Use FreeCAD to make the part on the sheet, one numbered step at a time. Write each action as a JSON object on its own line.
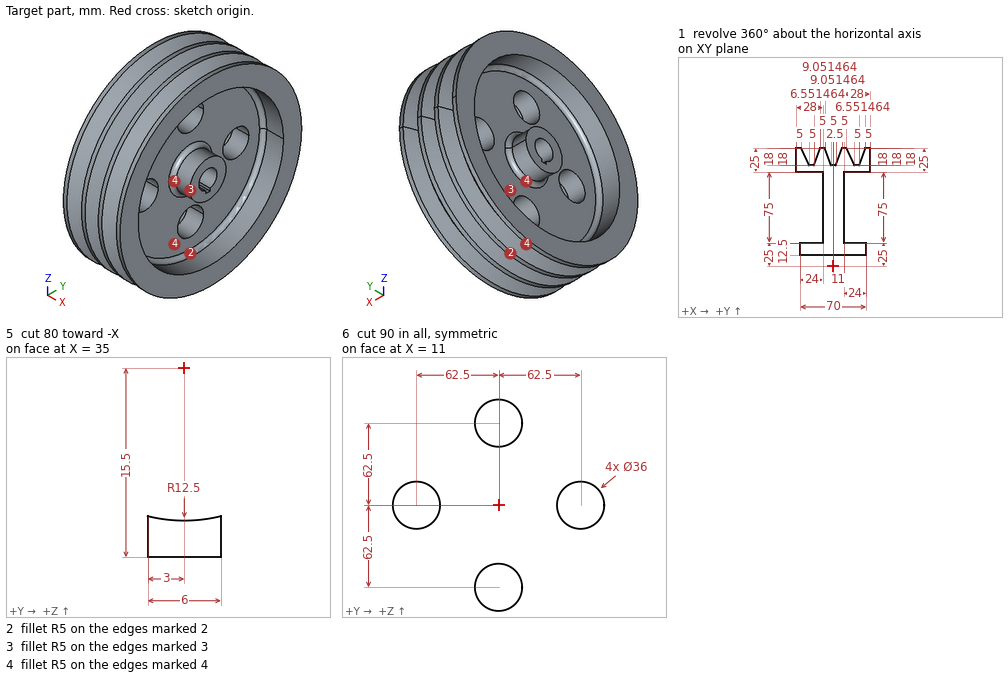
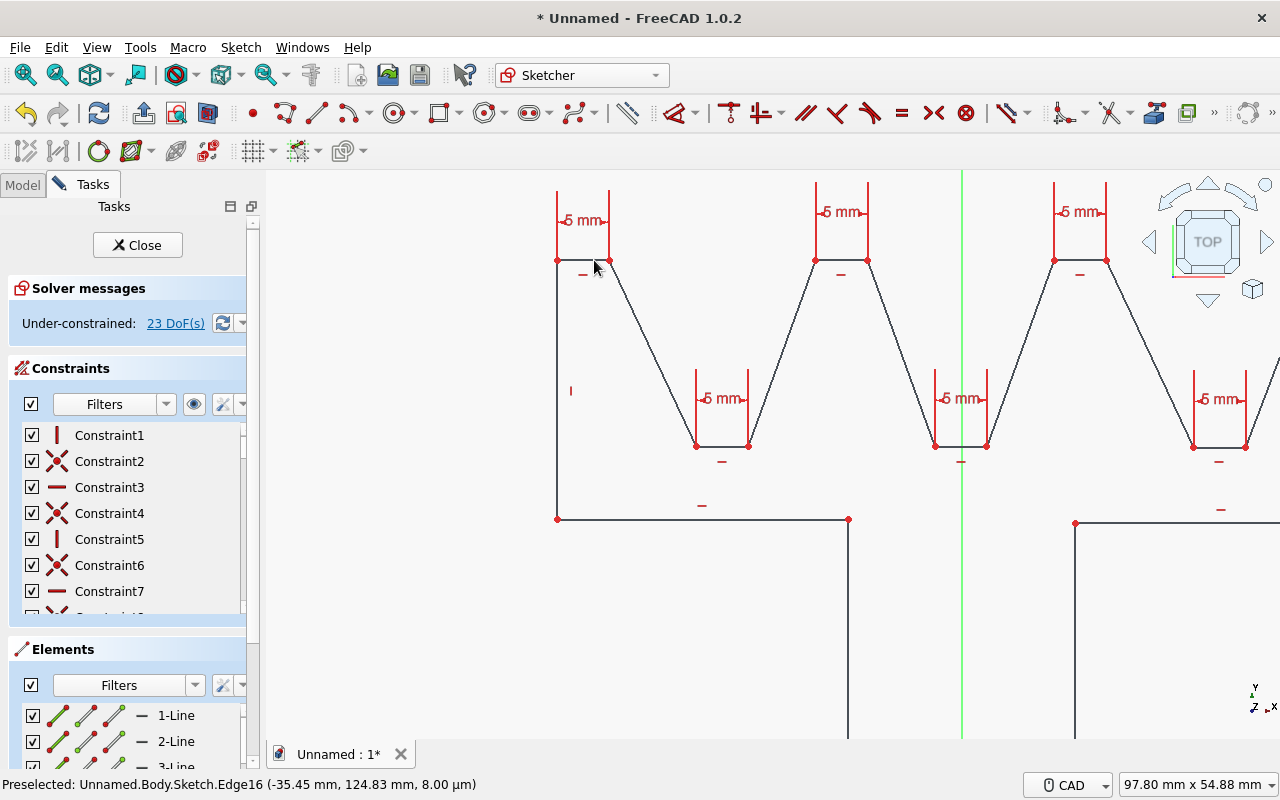
{"action": "scroll", "coordinate": [594, 260], "scroll_direction": "down", "scroll_amount": 6}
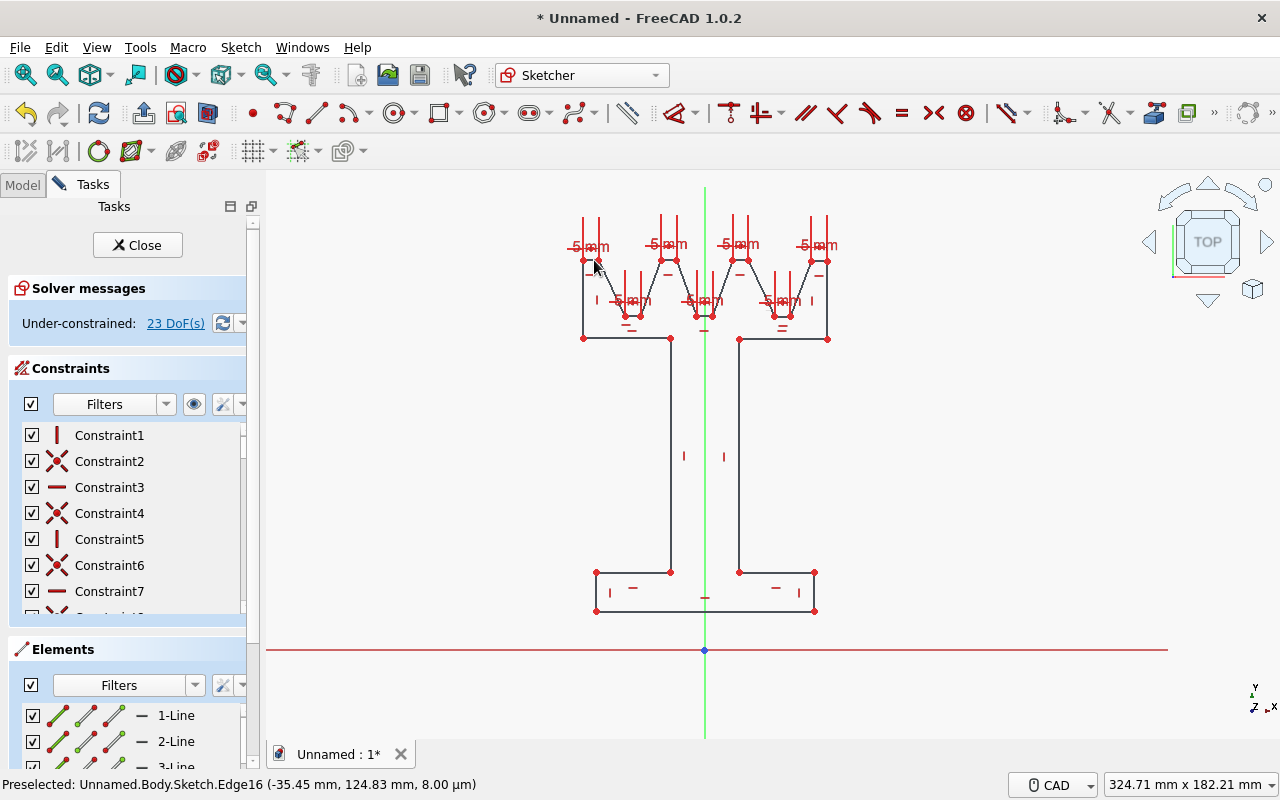
{"action": "left_click", "coordinate": [739, 386]}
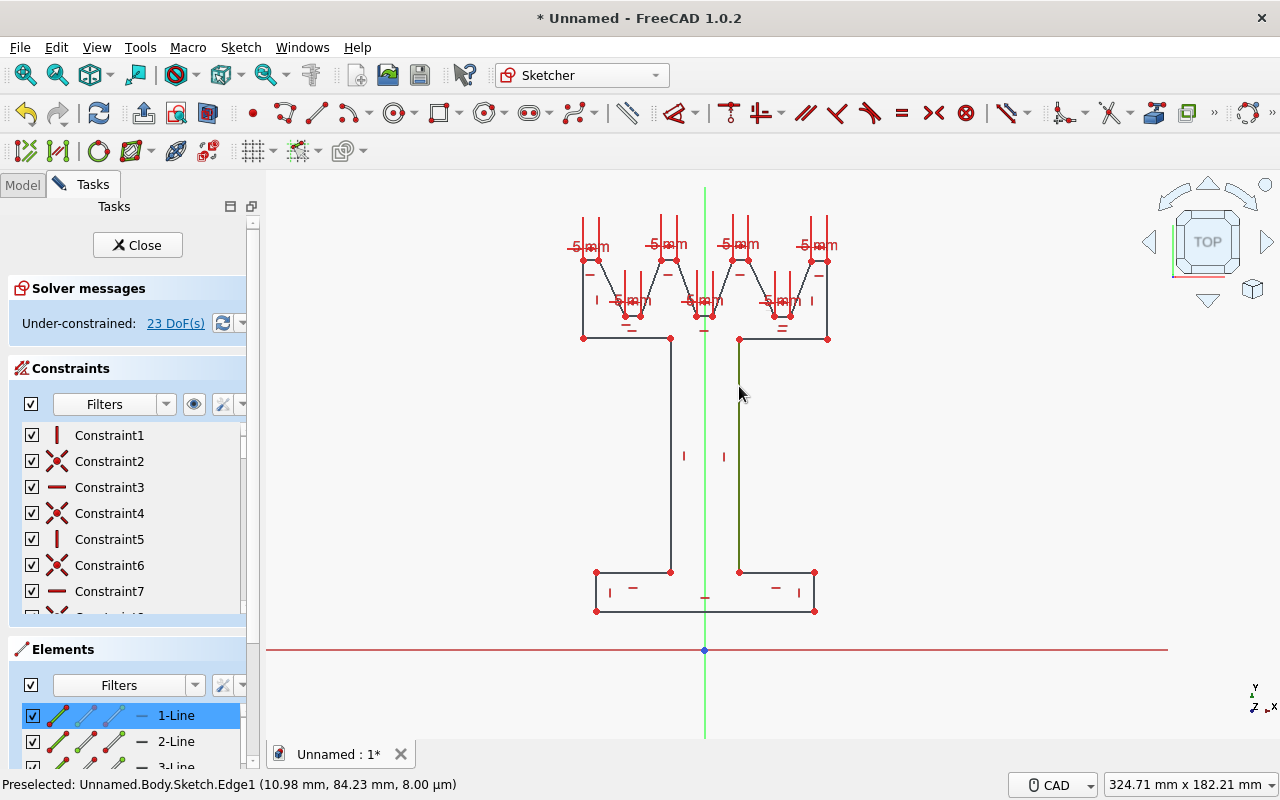
{"action": "left_click", "coordinate": [698, 114]}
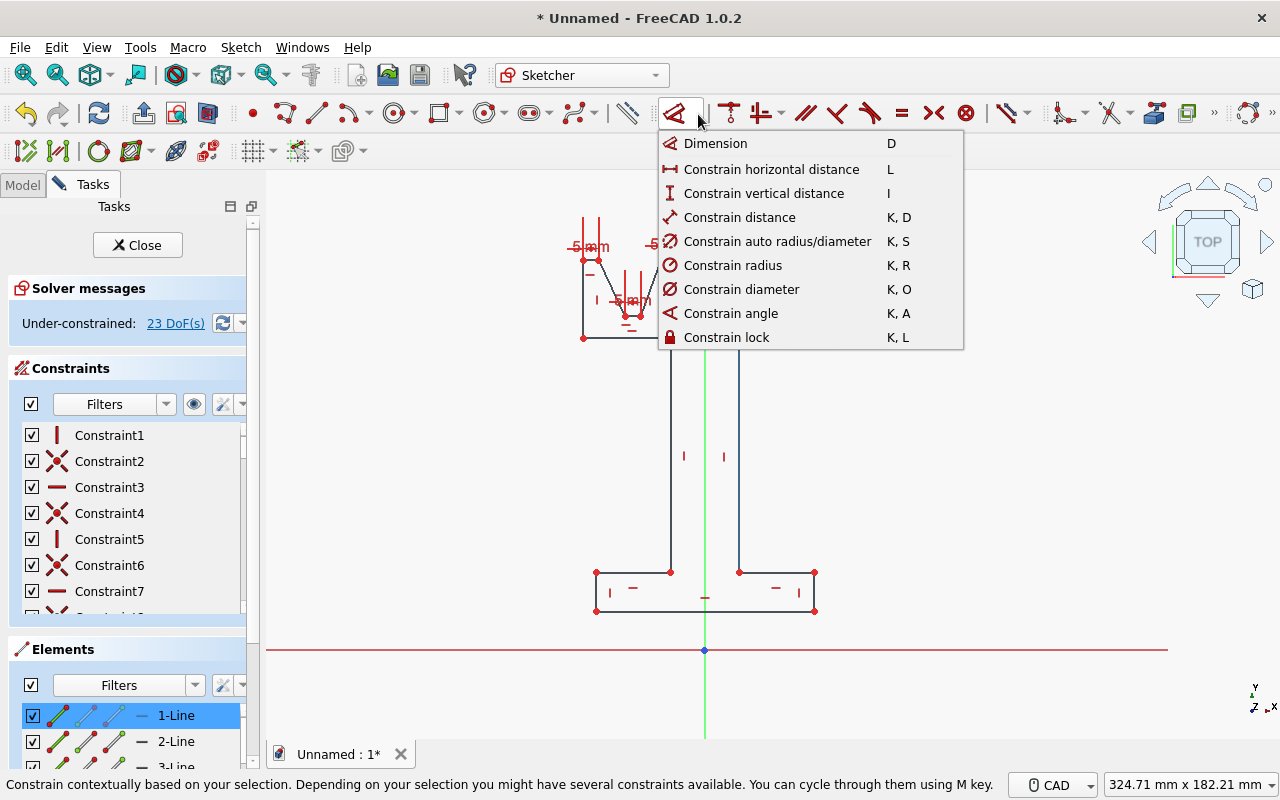
{"action": "left_click", "coordinate": [811, 193]}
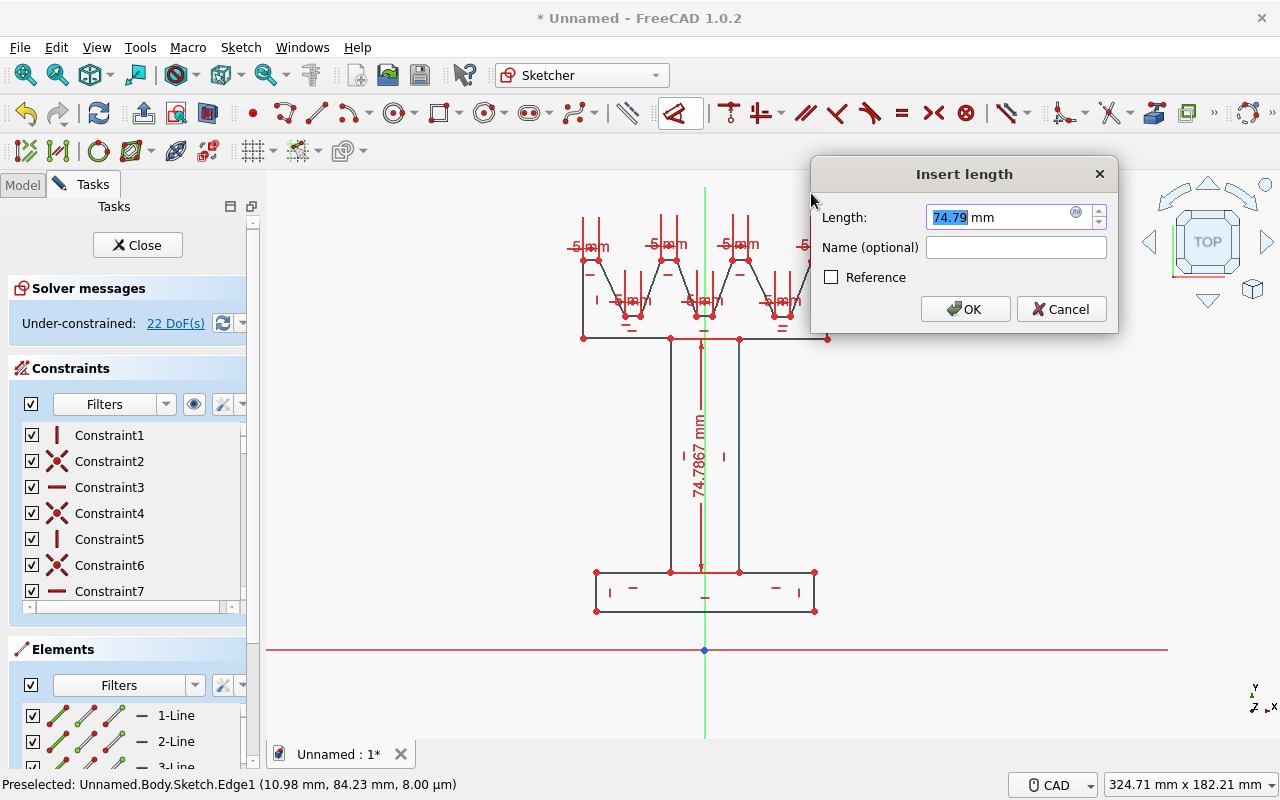
{"action": "type", "text": "75"}
{"action": "key", "text": "Return"}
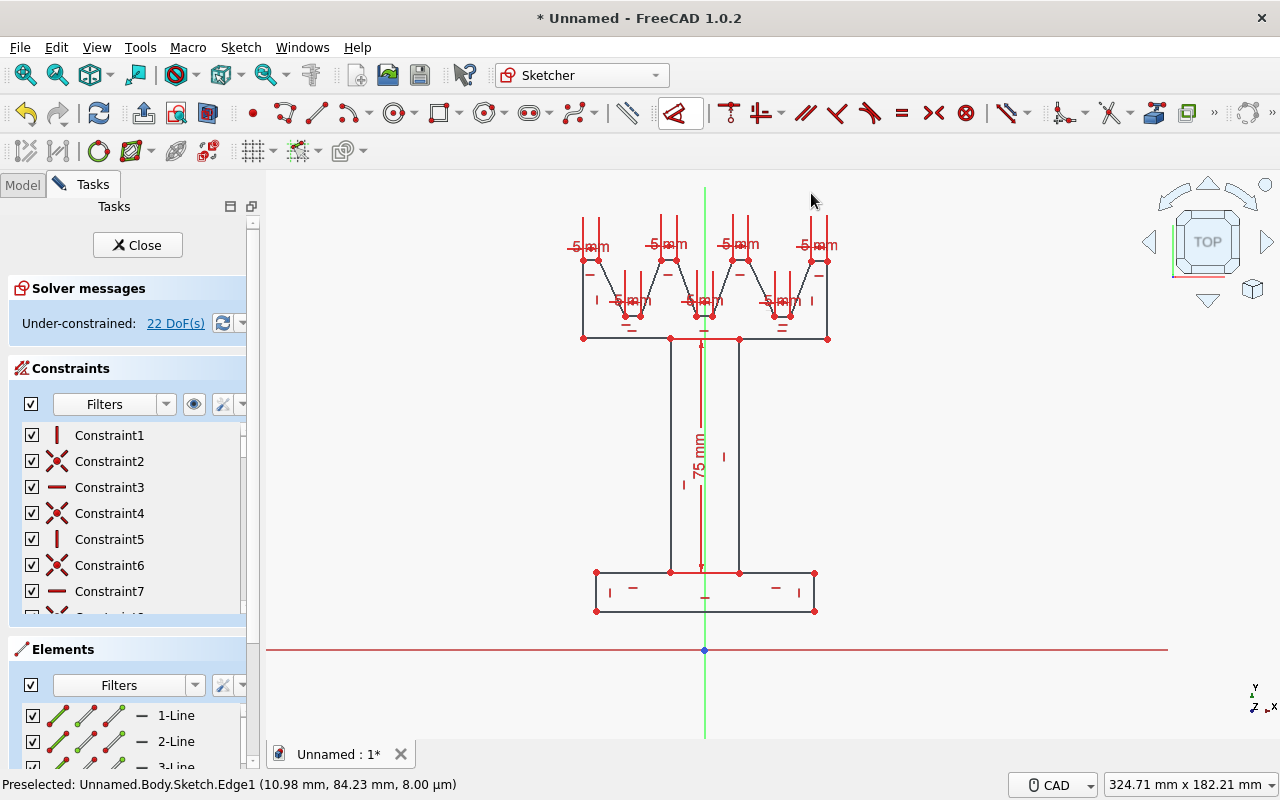
{"action": "left_click", "coordinate": [766, 339]}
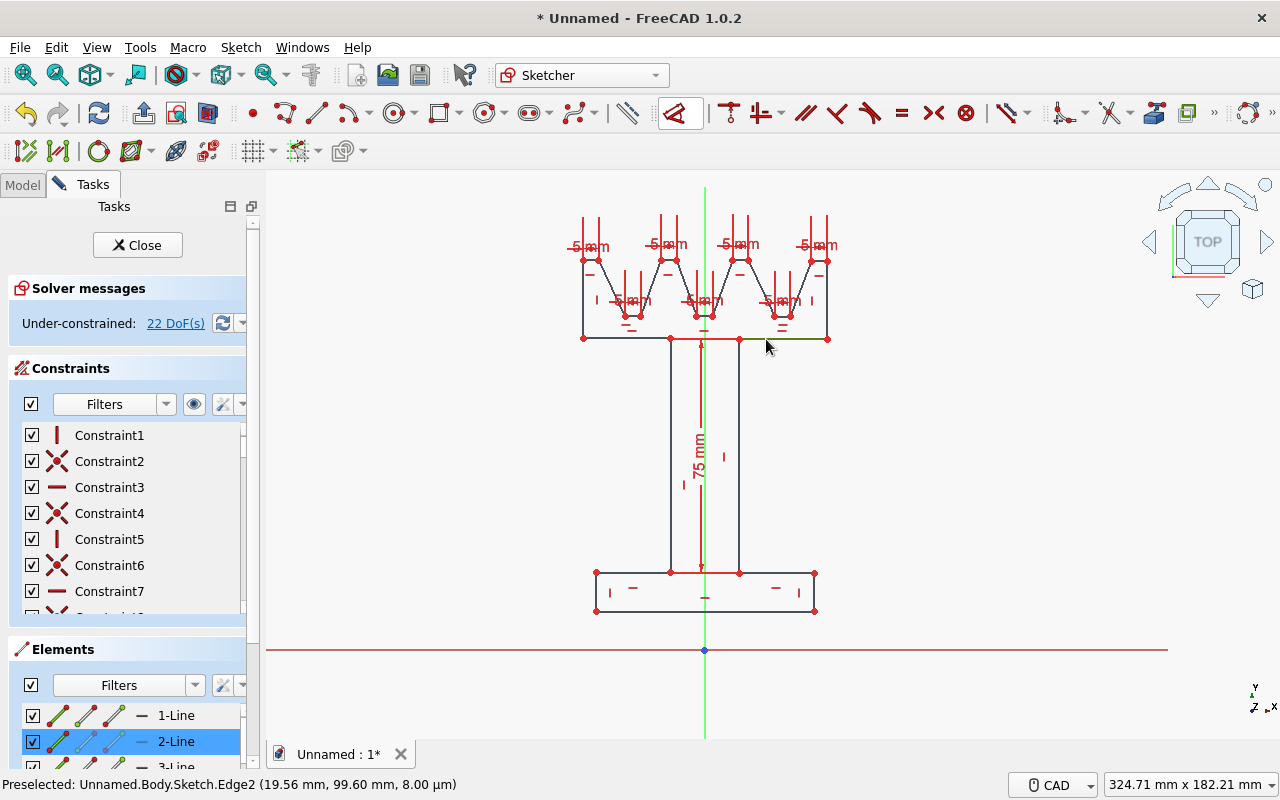
{"action": "key", "text": "l"}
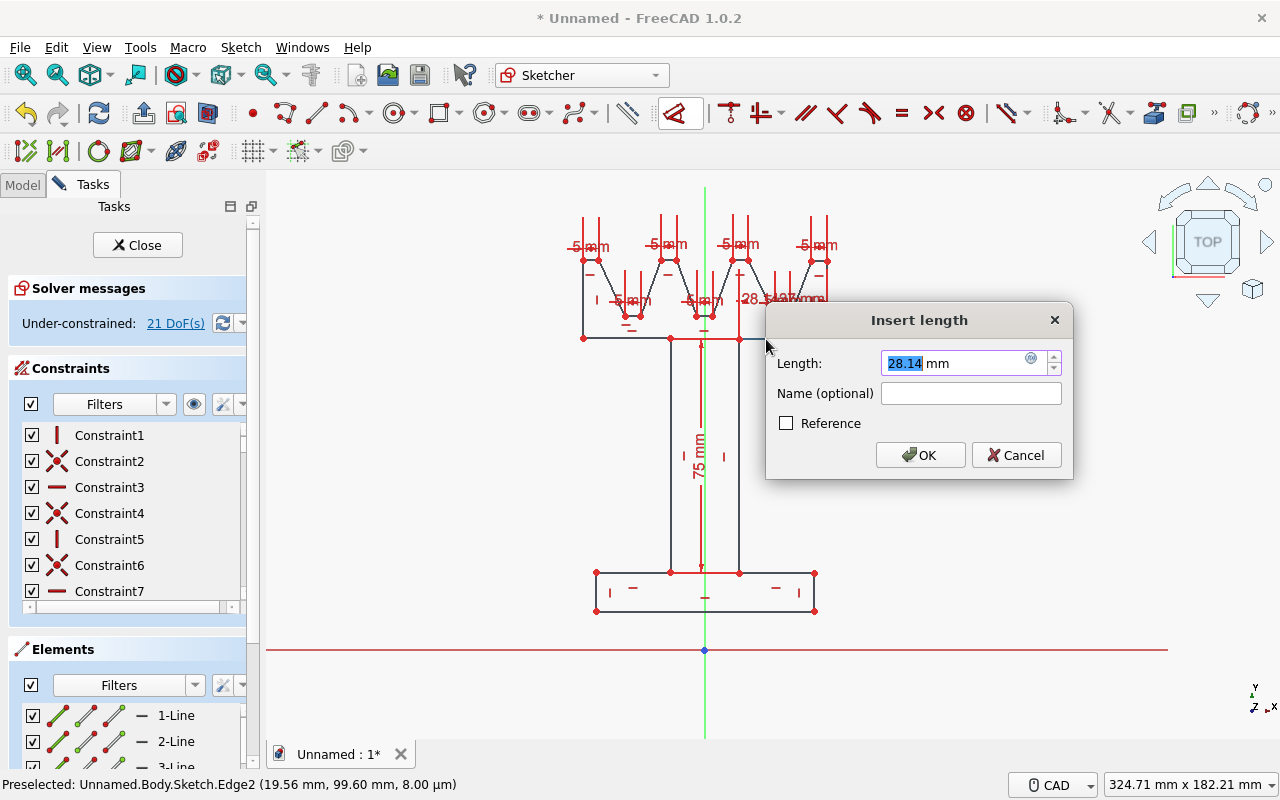
{"action": "type", "text": "28"}
{"action": "key", "text": "Return"}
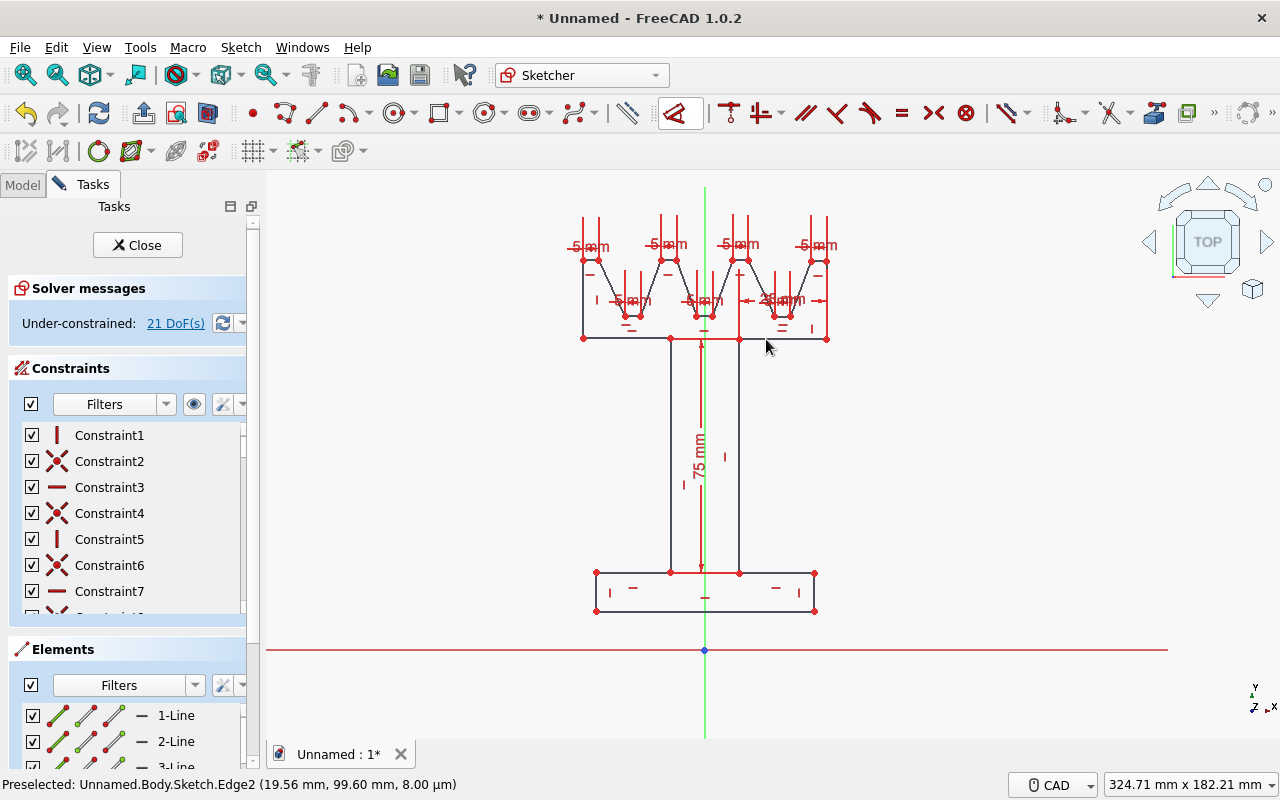
{"action": "left_click", "coordinate": [827, 316]}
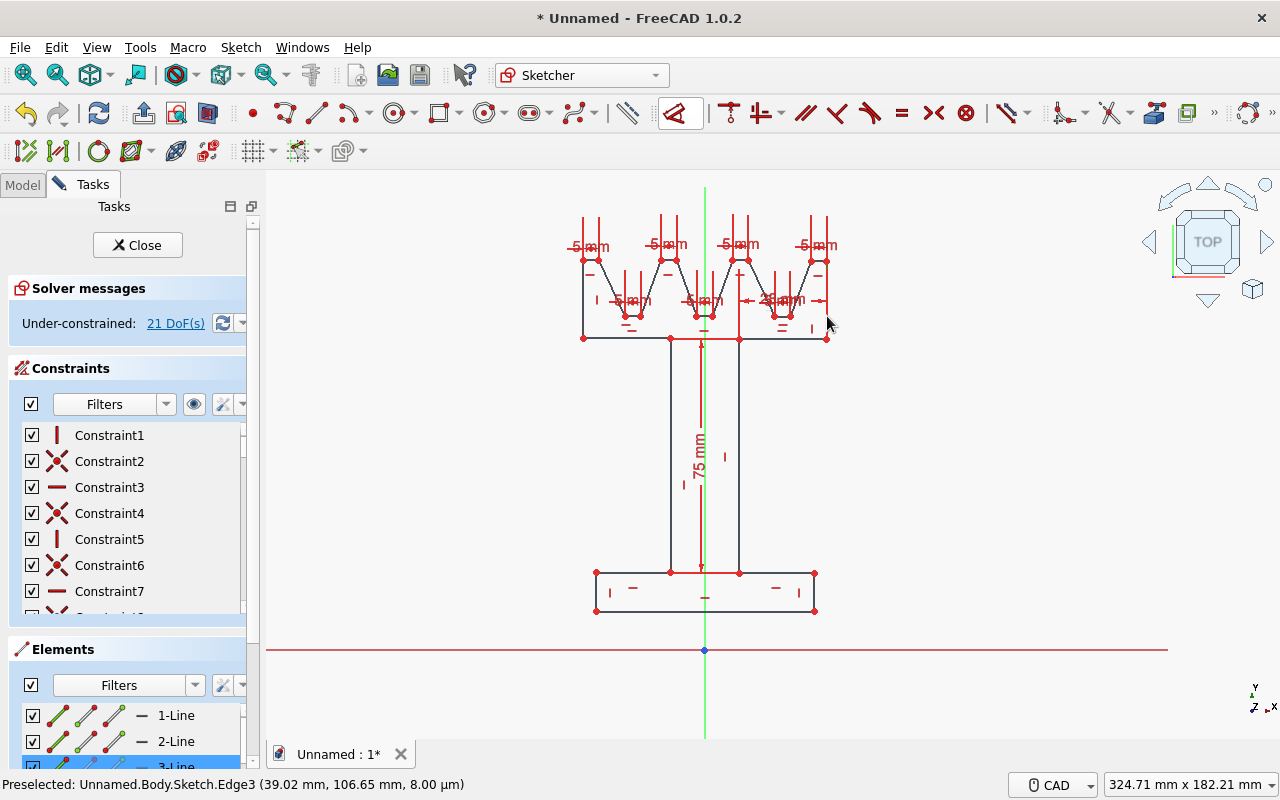
{"action": "left_click", "coordinate": [698, 114]}